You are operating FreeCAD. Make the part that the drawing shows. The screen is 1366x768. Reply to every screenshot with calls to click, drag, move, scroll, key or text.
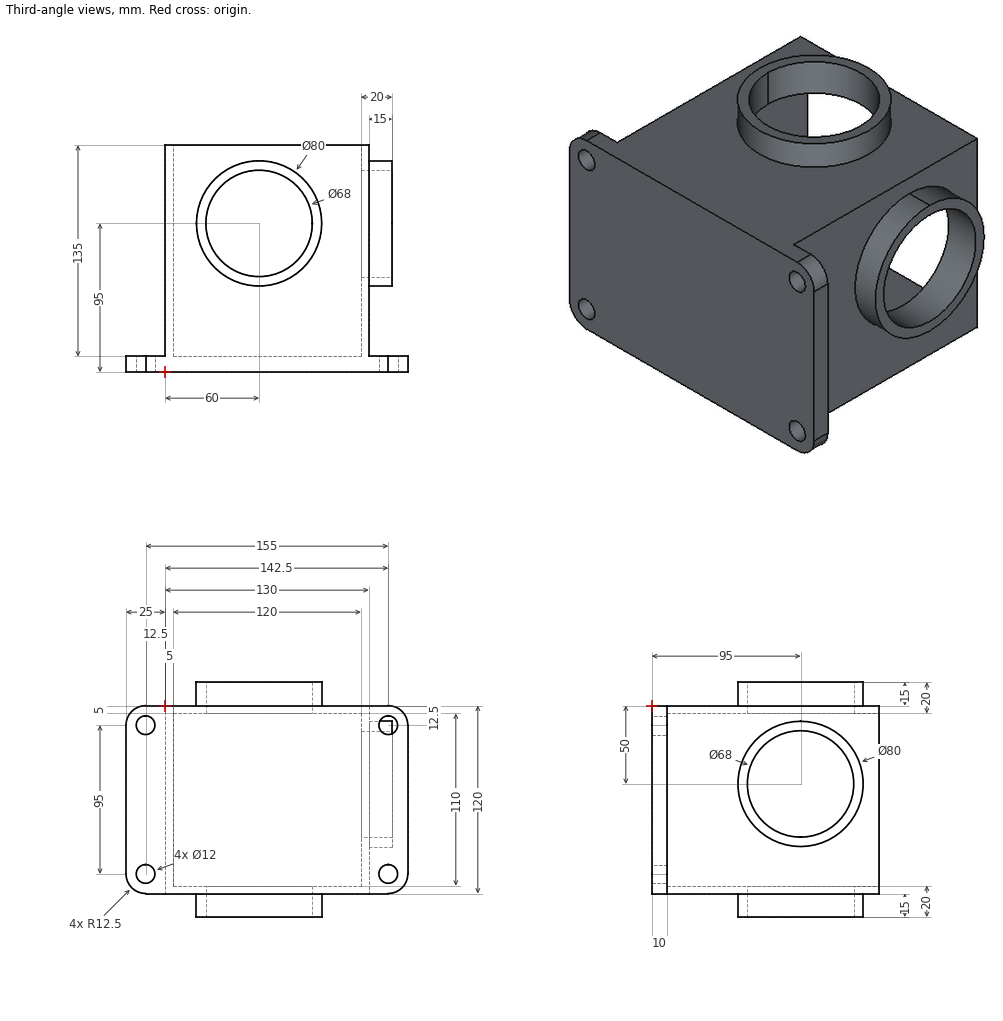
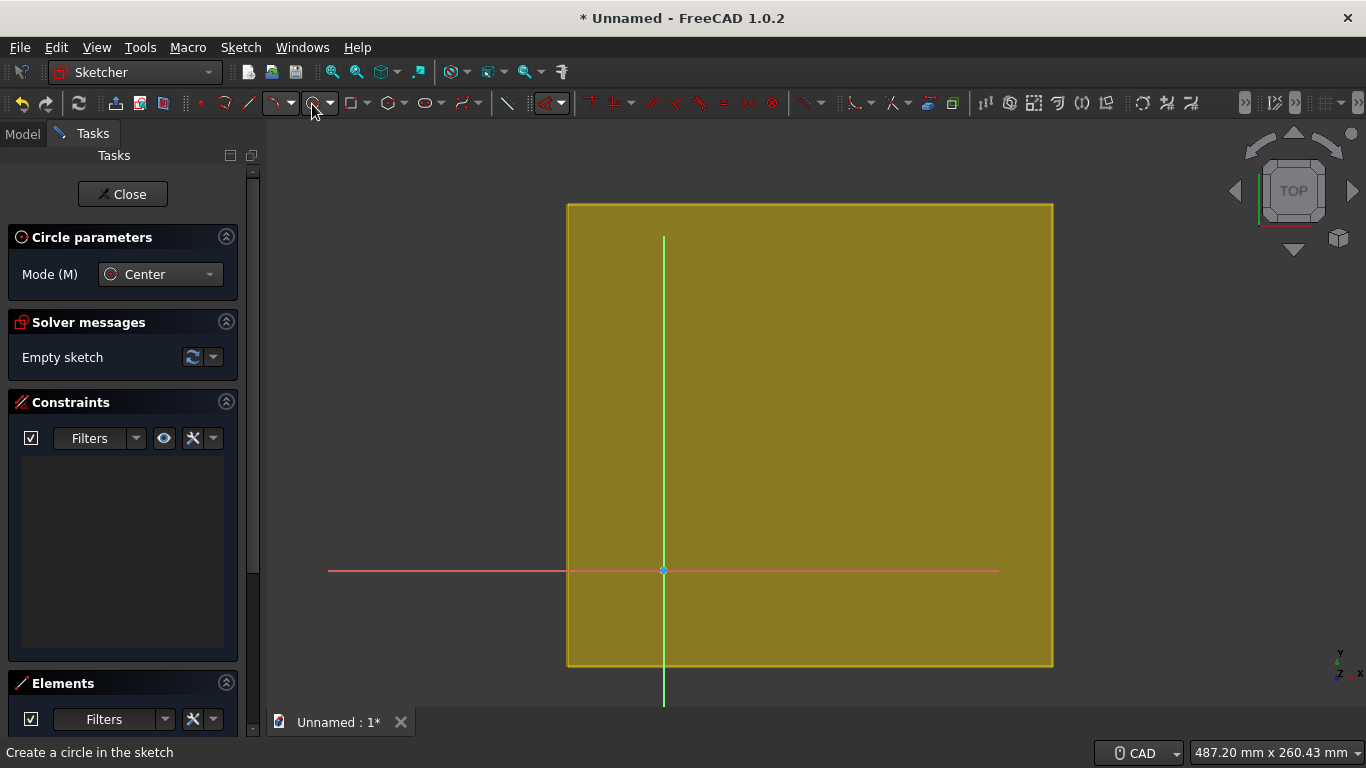
click(799, 356)
move(863, 293)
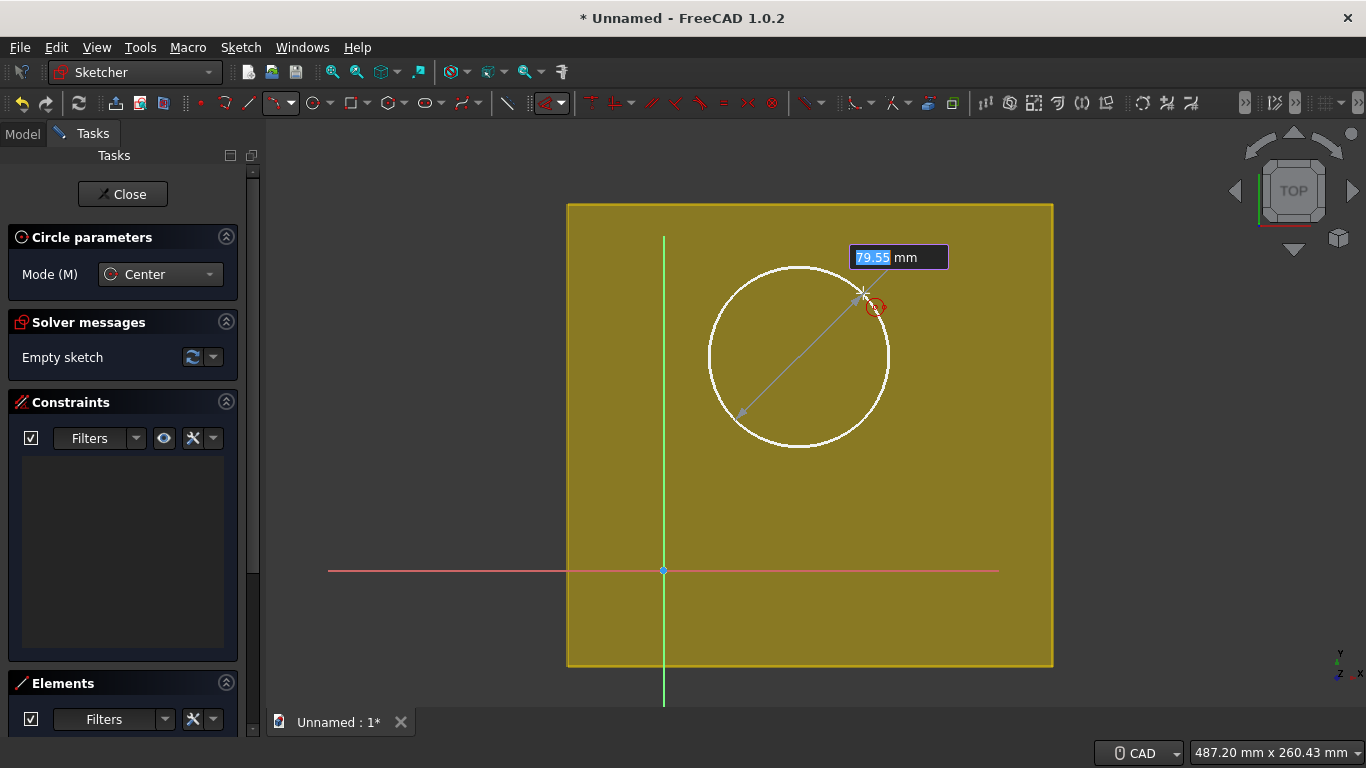
text(80)
key(Return)
key(Escape)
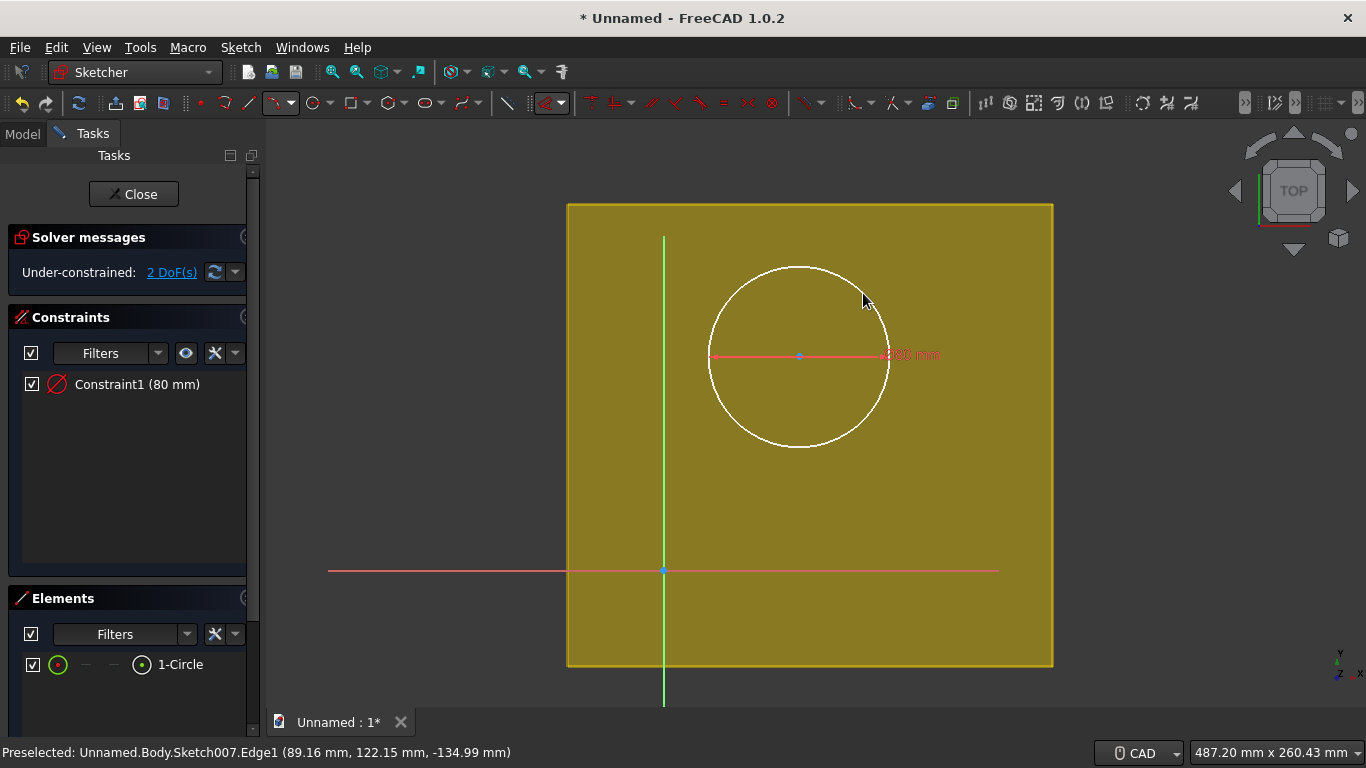
click(799, 357)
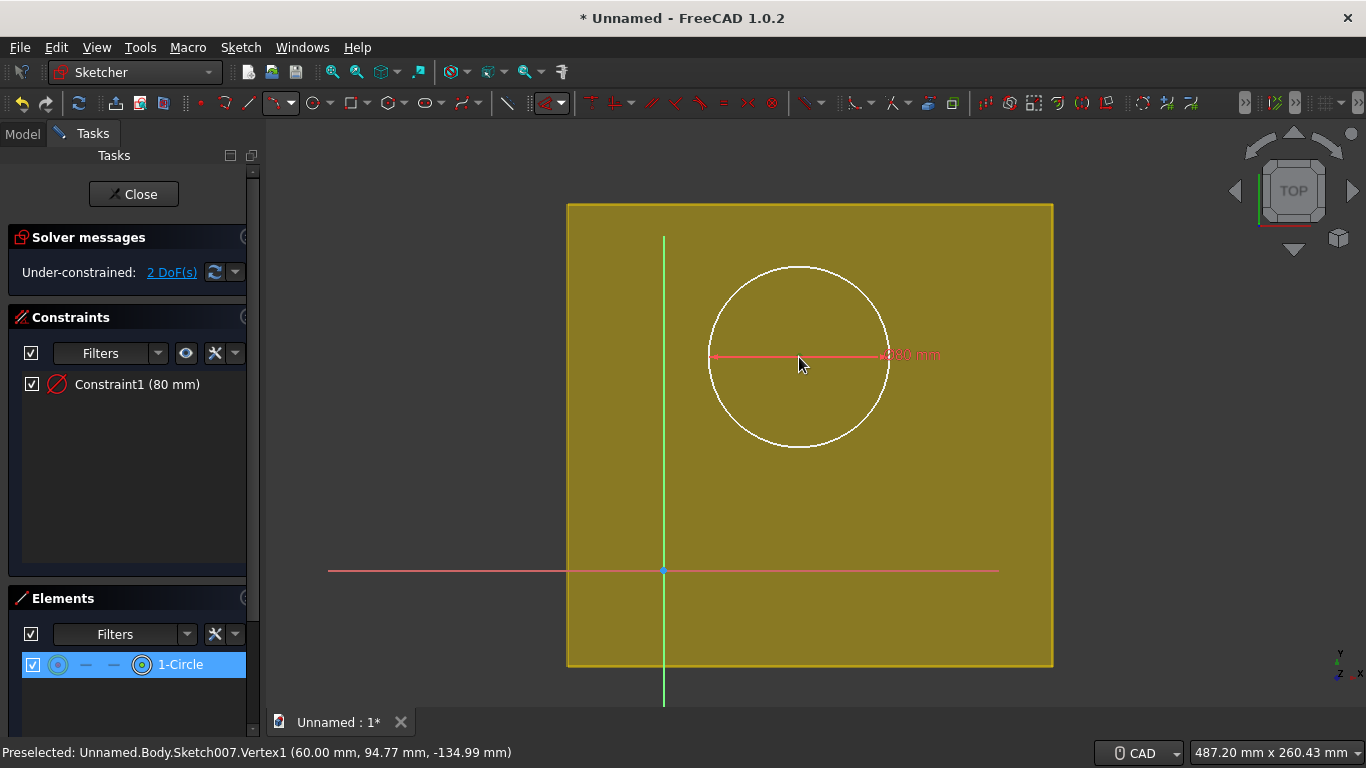
key(l)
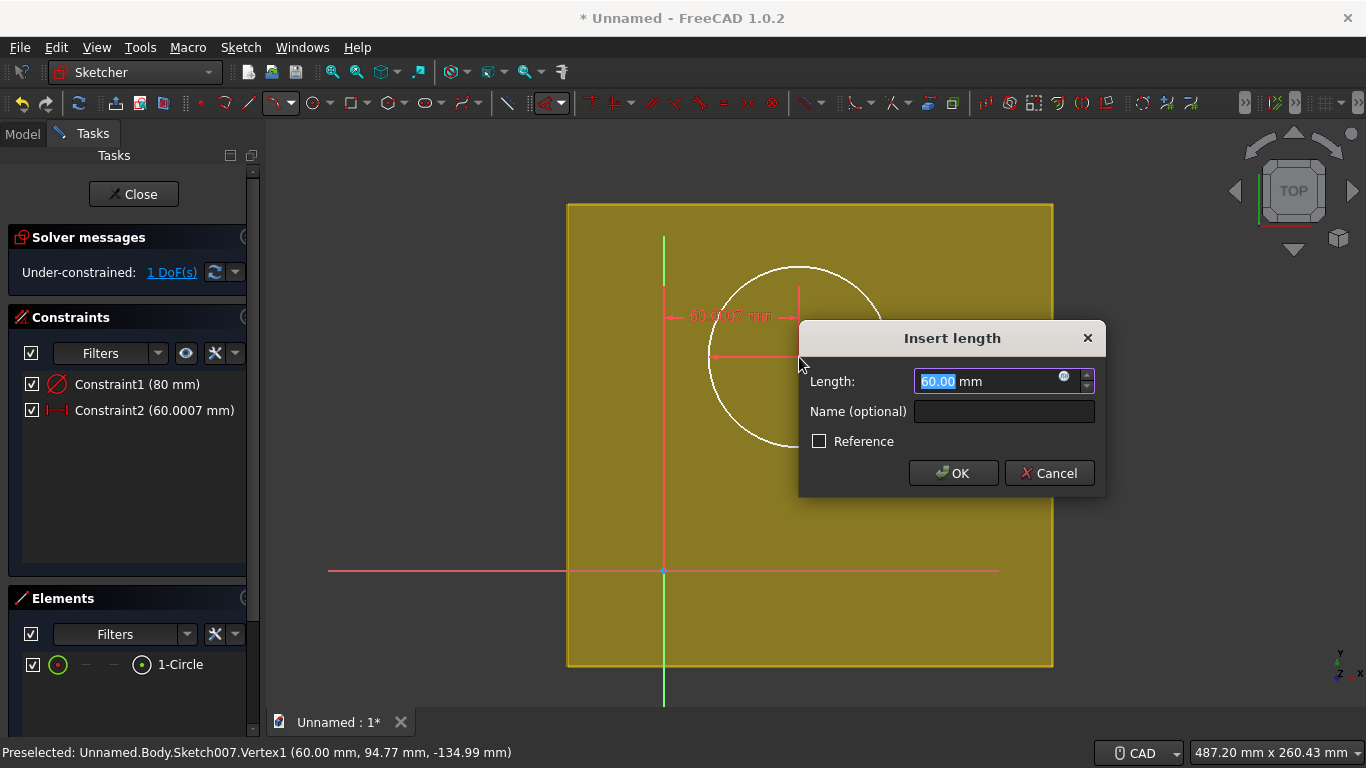
text(60)
key(Return)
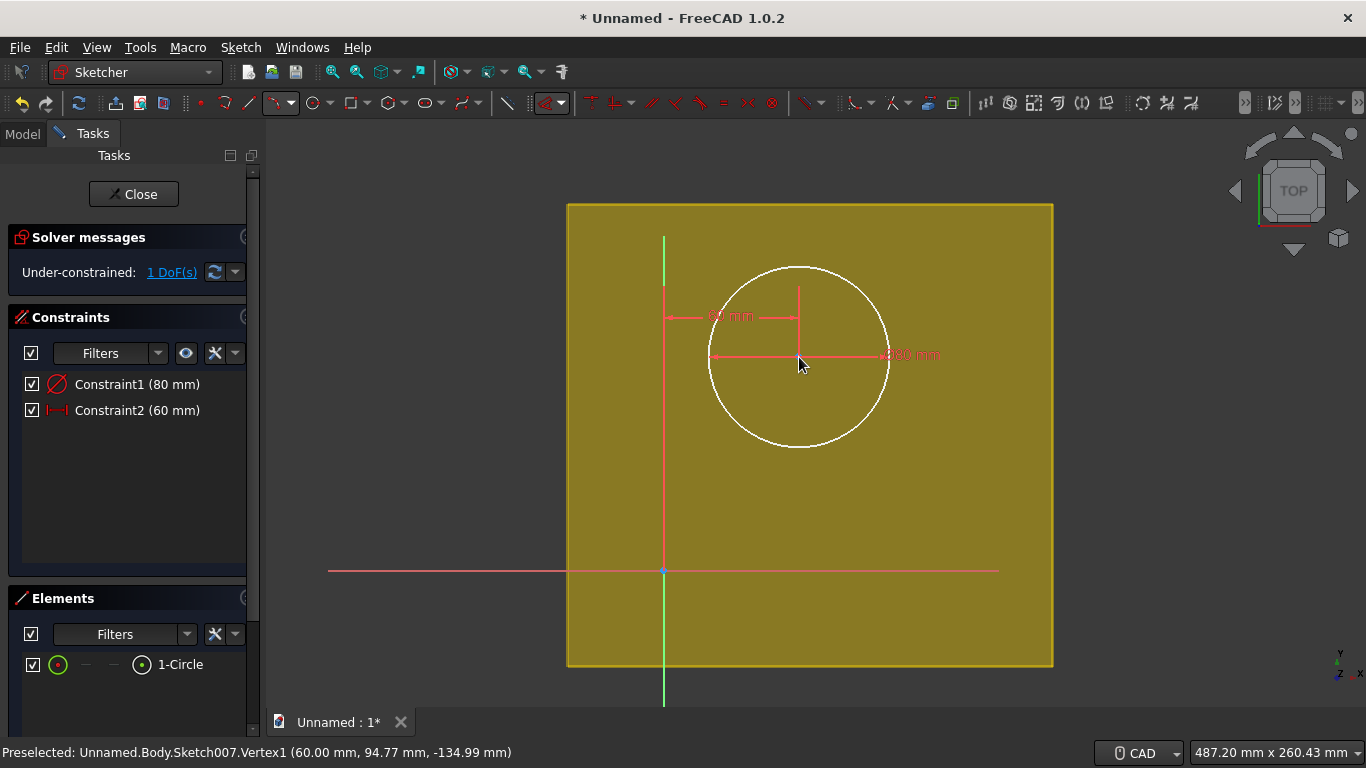
click(799, 357)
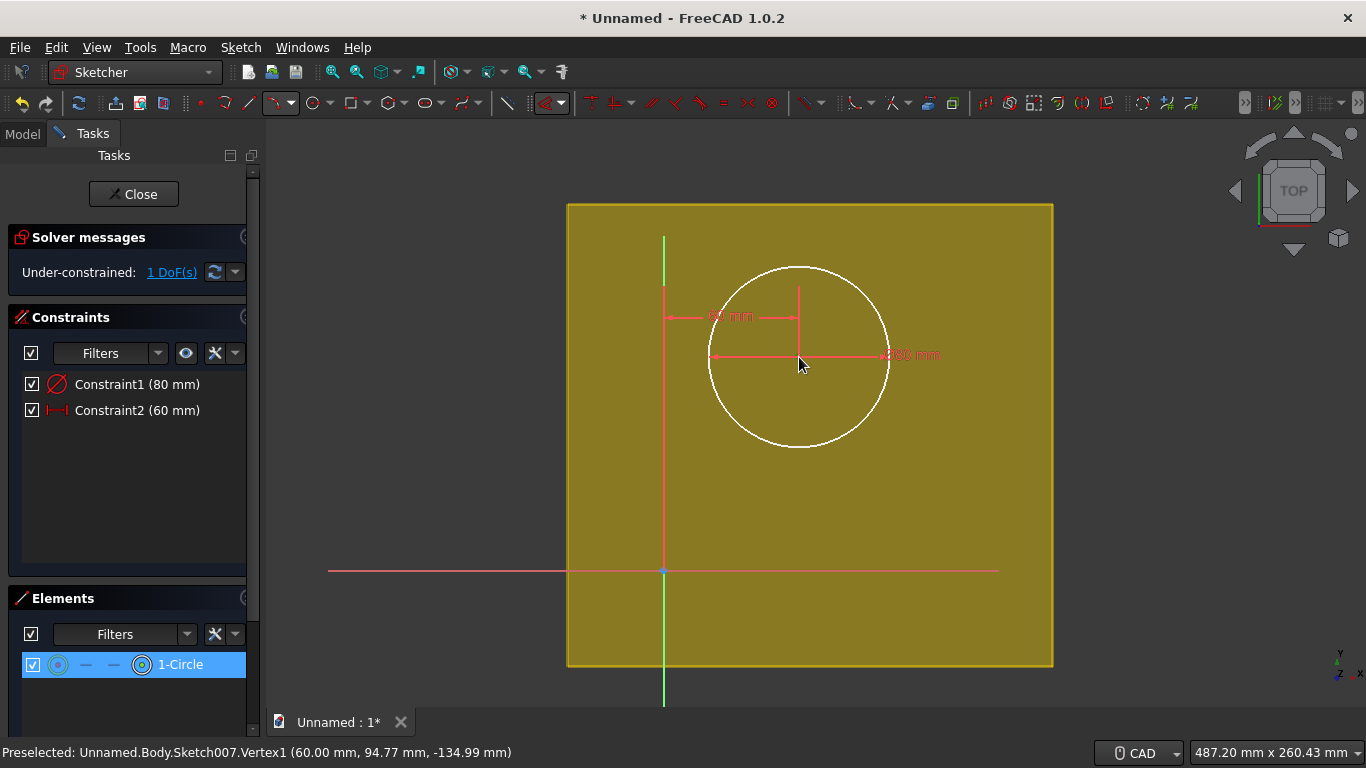
click(564, 104)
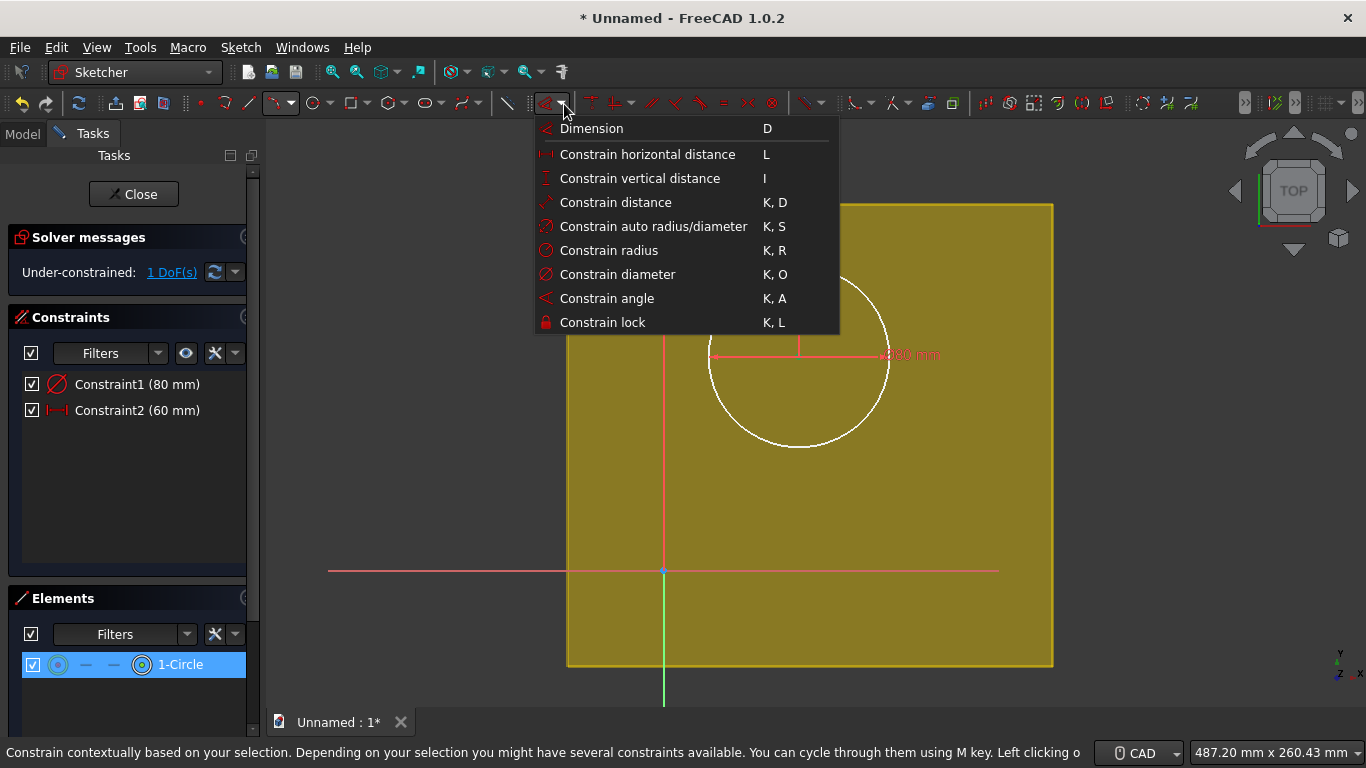
click(687, 178)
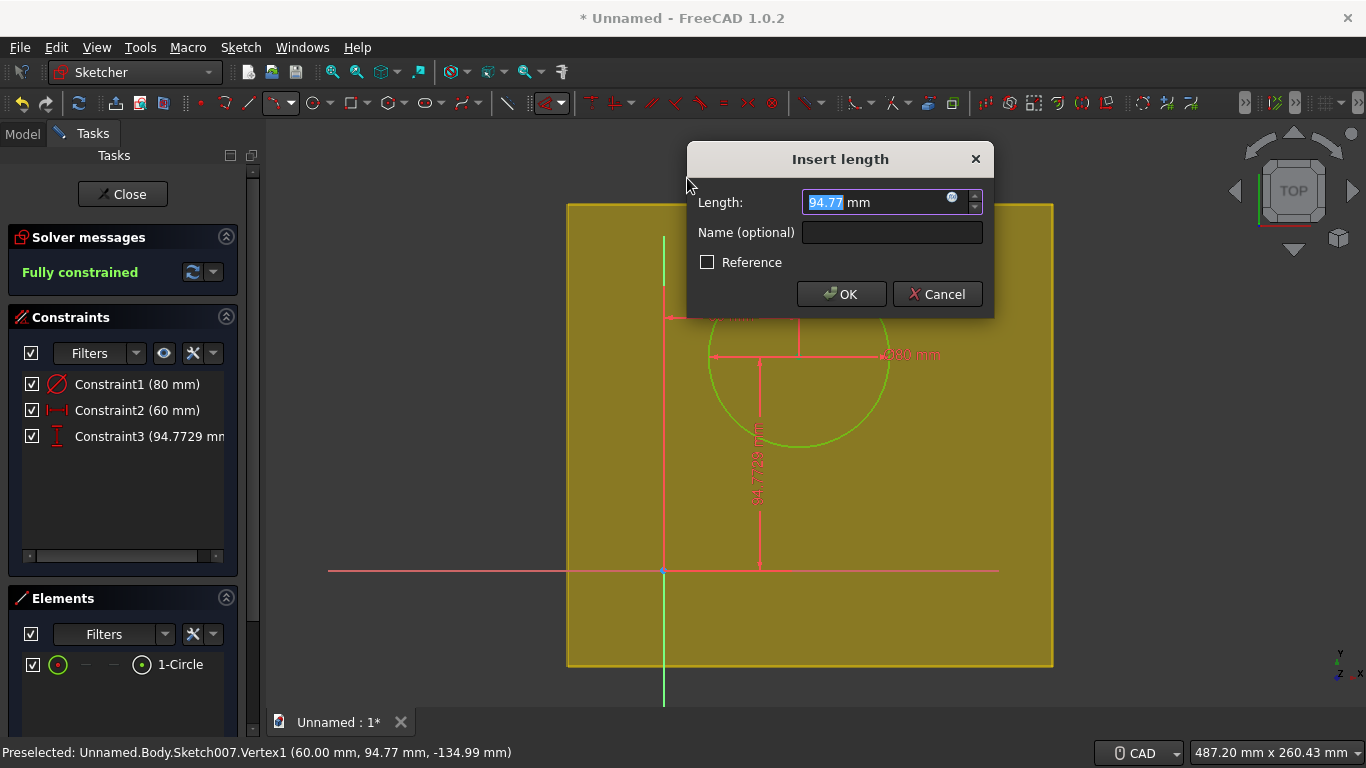
text(95)
key(Return)